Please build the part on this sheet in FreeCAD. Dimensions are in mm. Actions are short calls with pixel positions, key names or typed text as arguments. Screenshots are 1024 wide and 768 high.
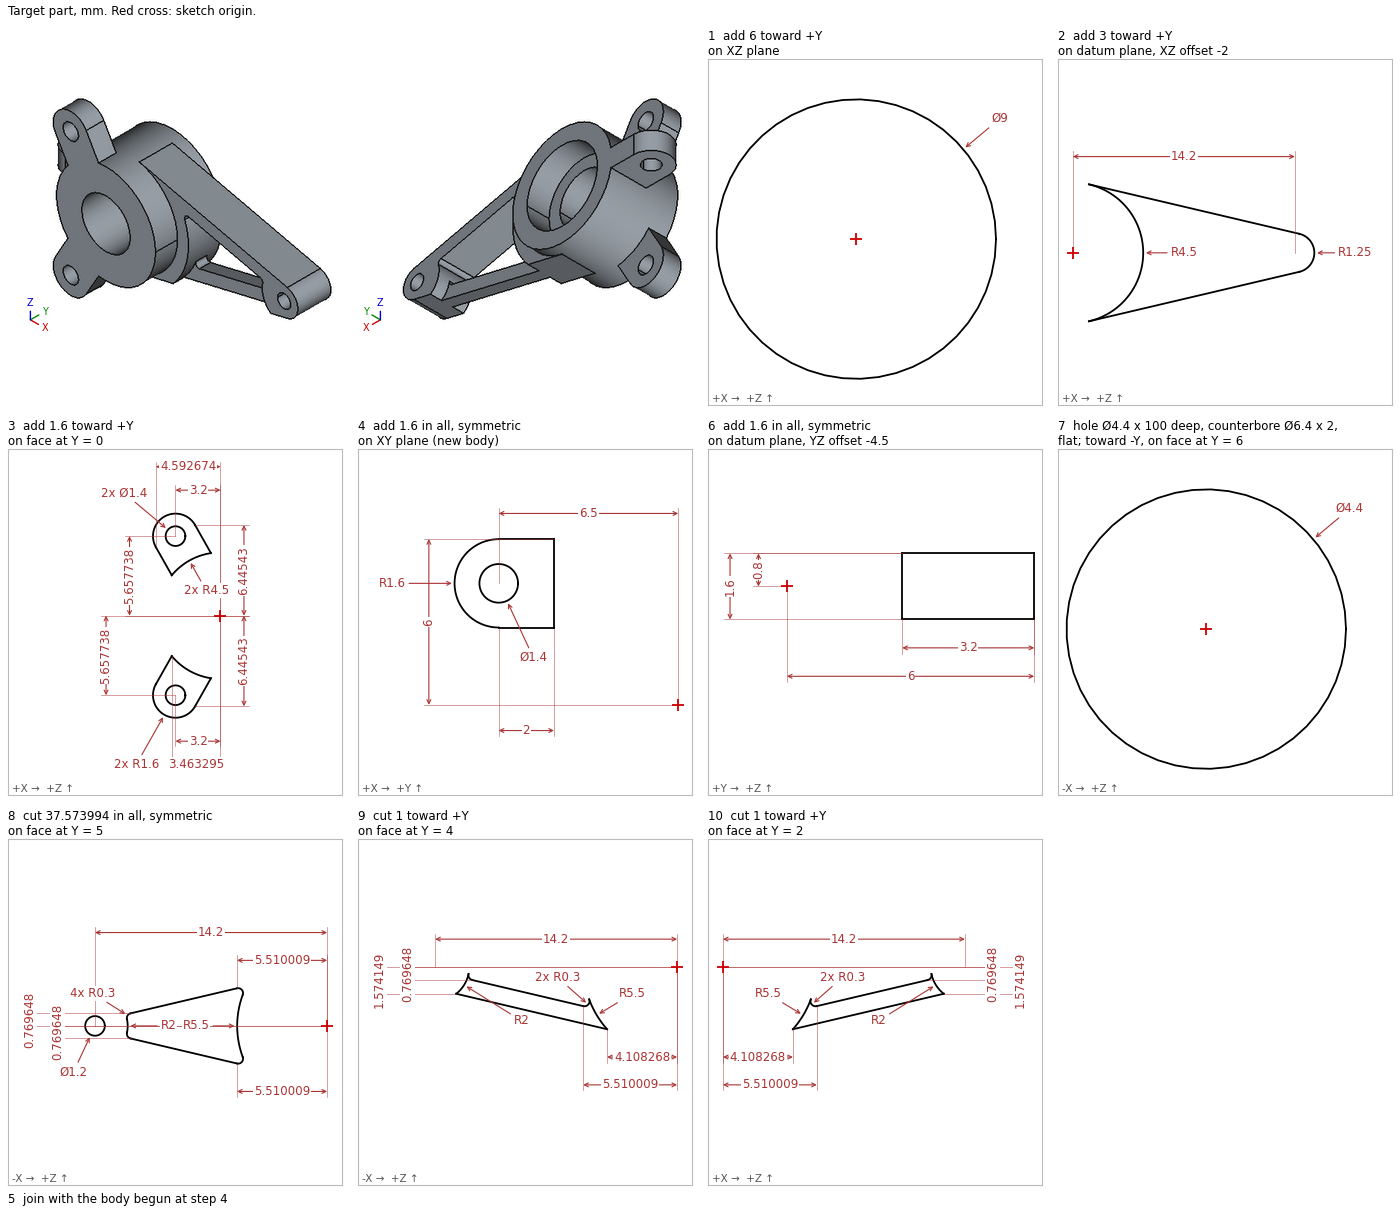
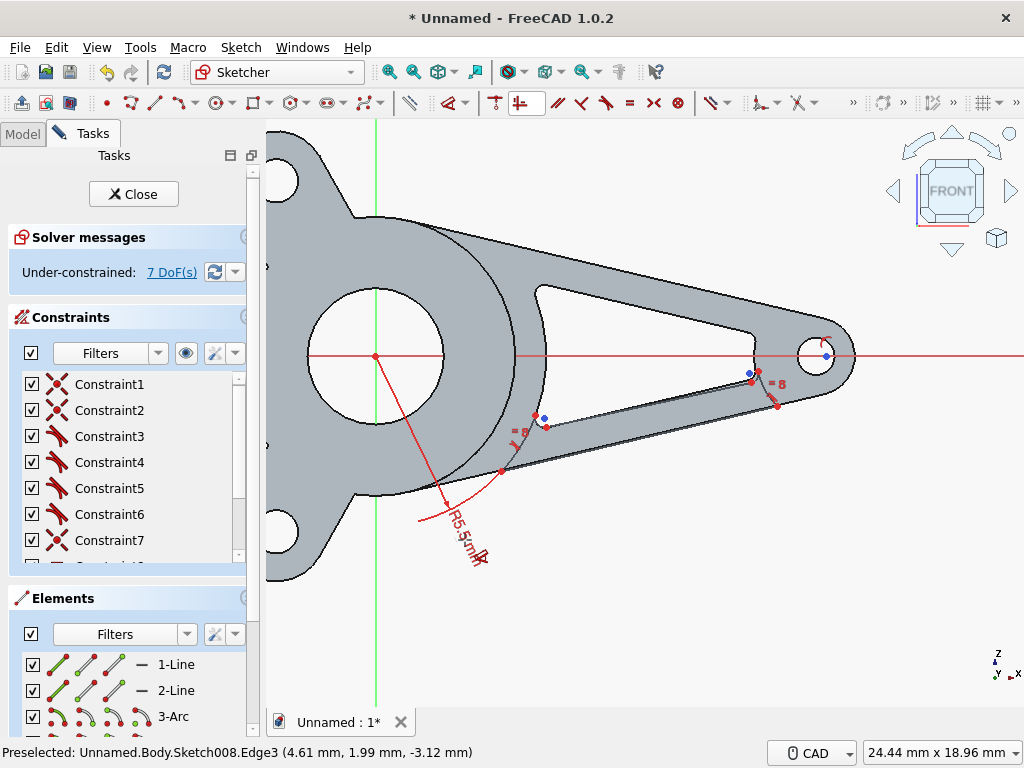
scroll(541, 427, up, 8)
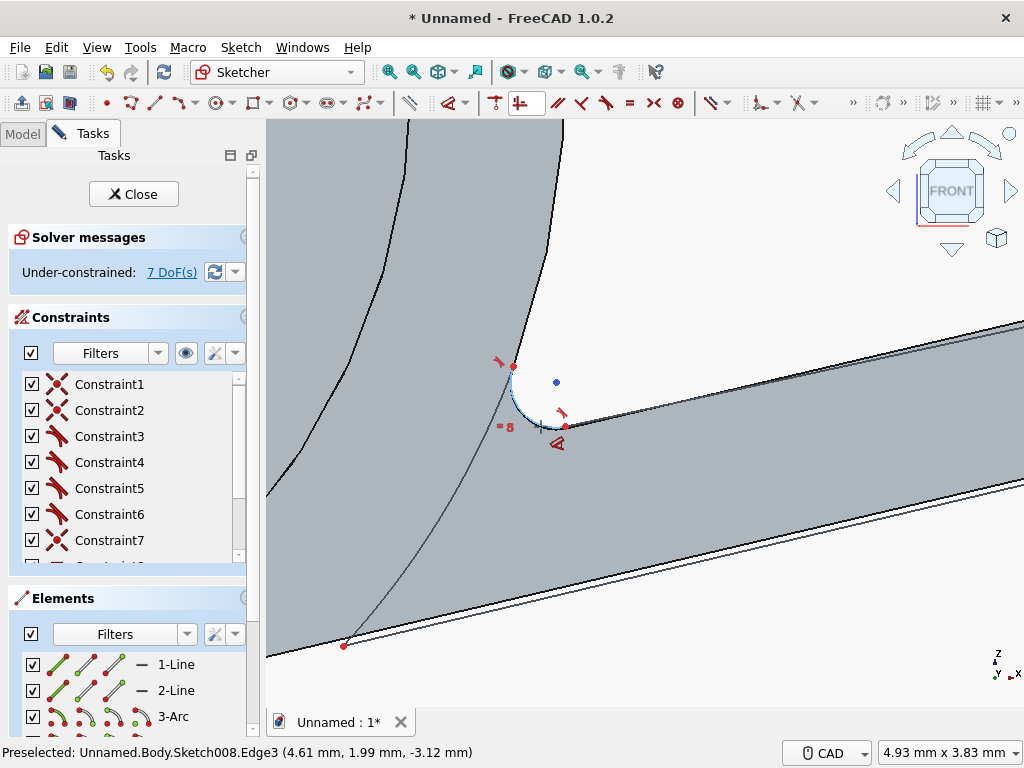
click(537, 424)
click(524, 453)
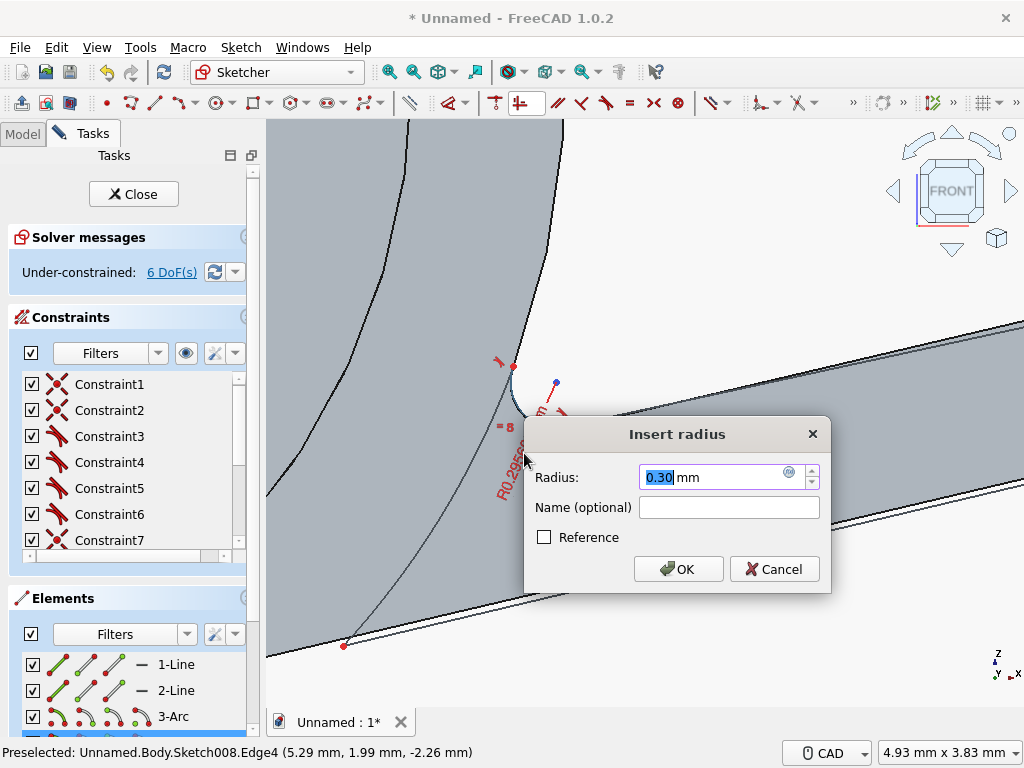
text(0.3)
key(Return)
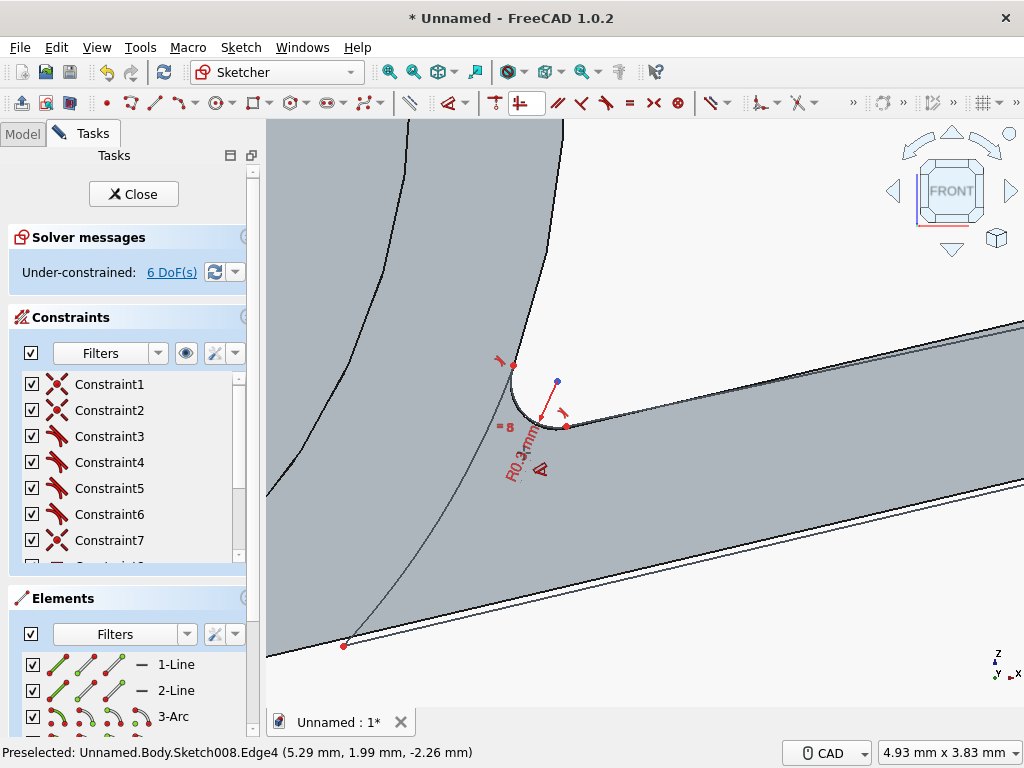
scroll(541, 427, down, 8)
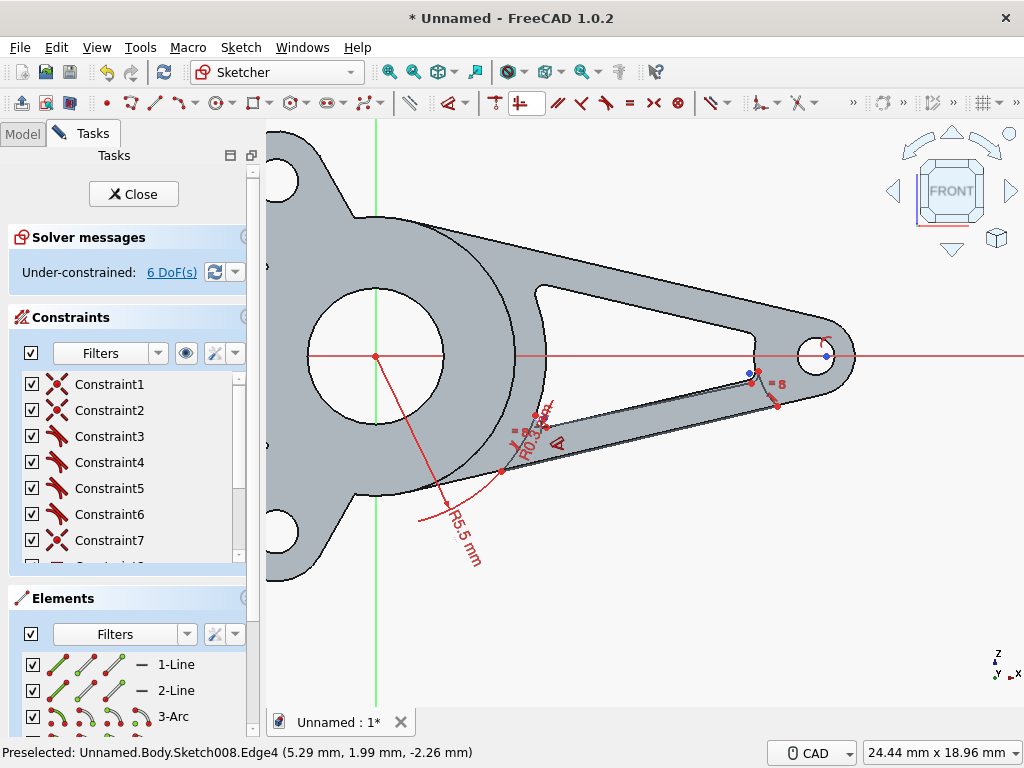
scroll(762, 383, up, 4)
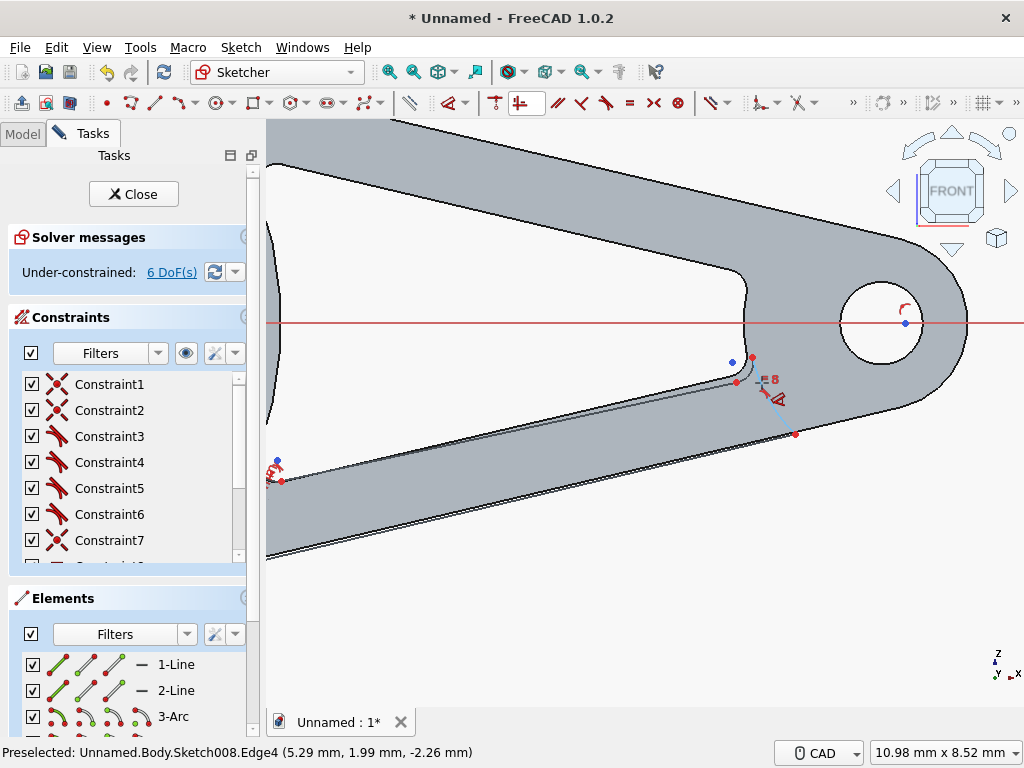
click(761, 383)
click(718, 303)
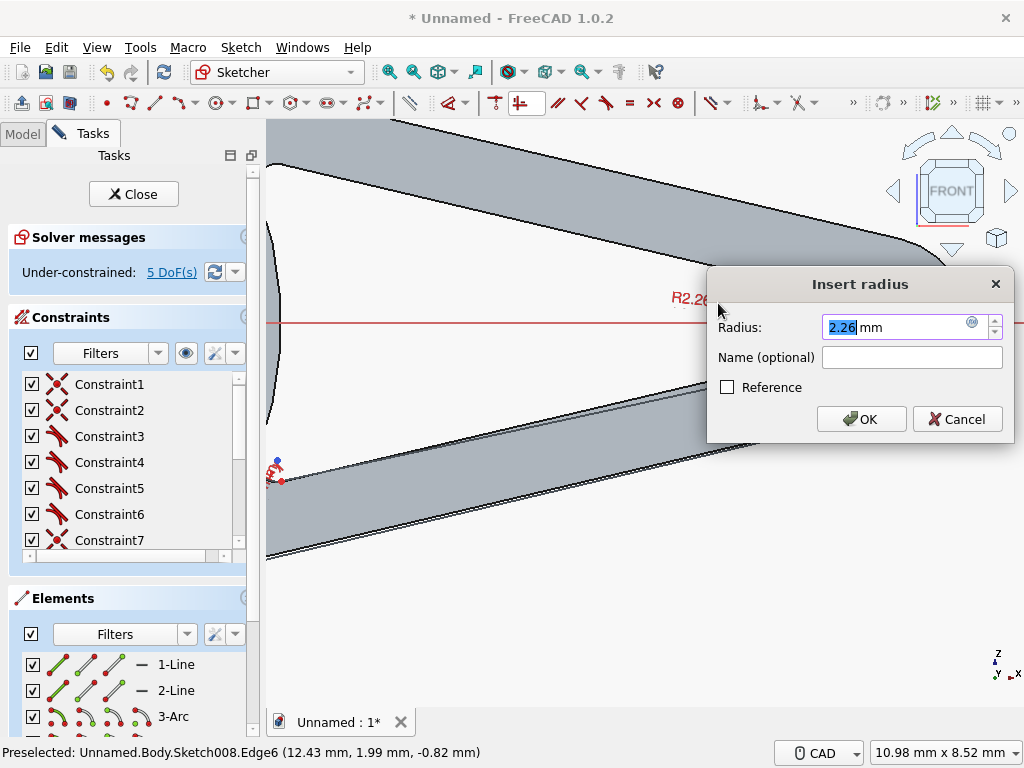
text(2)
key(Return)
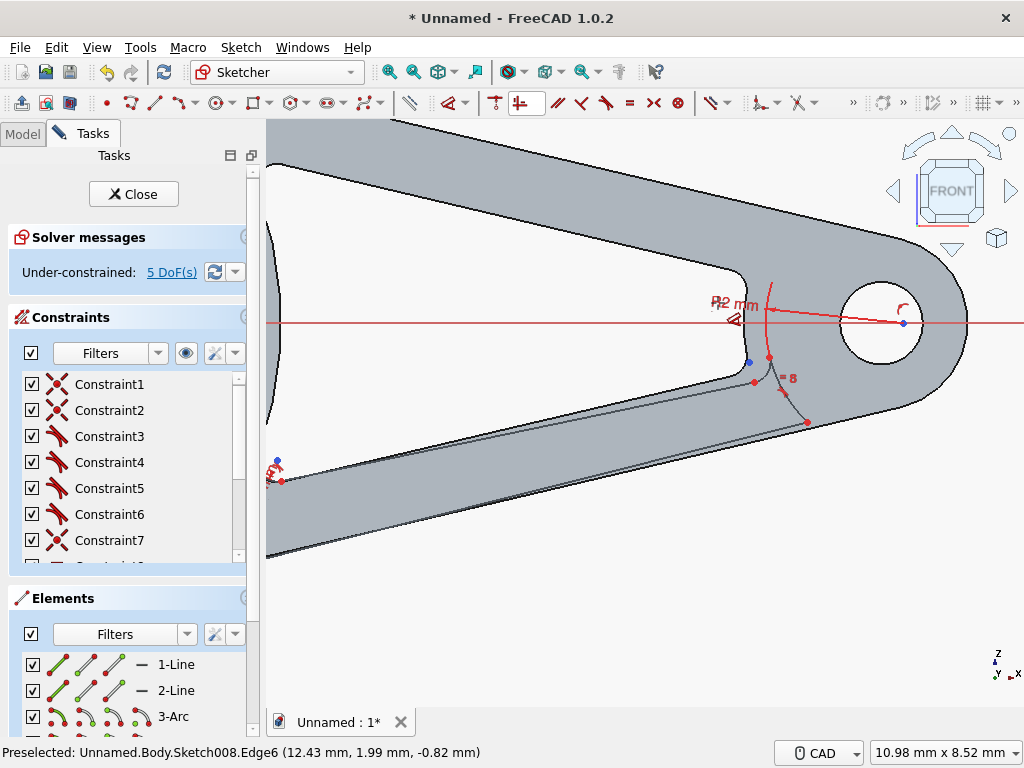
scroll(762, 383, down, 4)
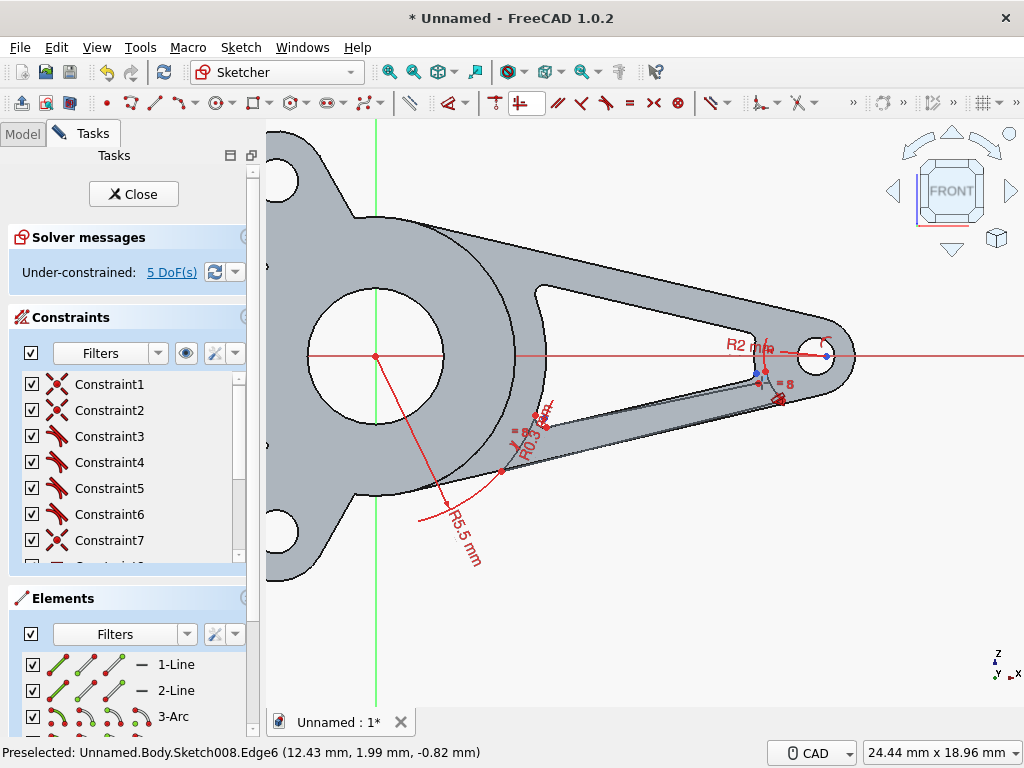
click(826, 356)
click(601, 322)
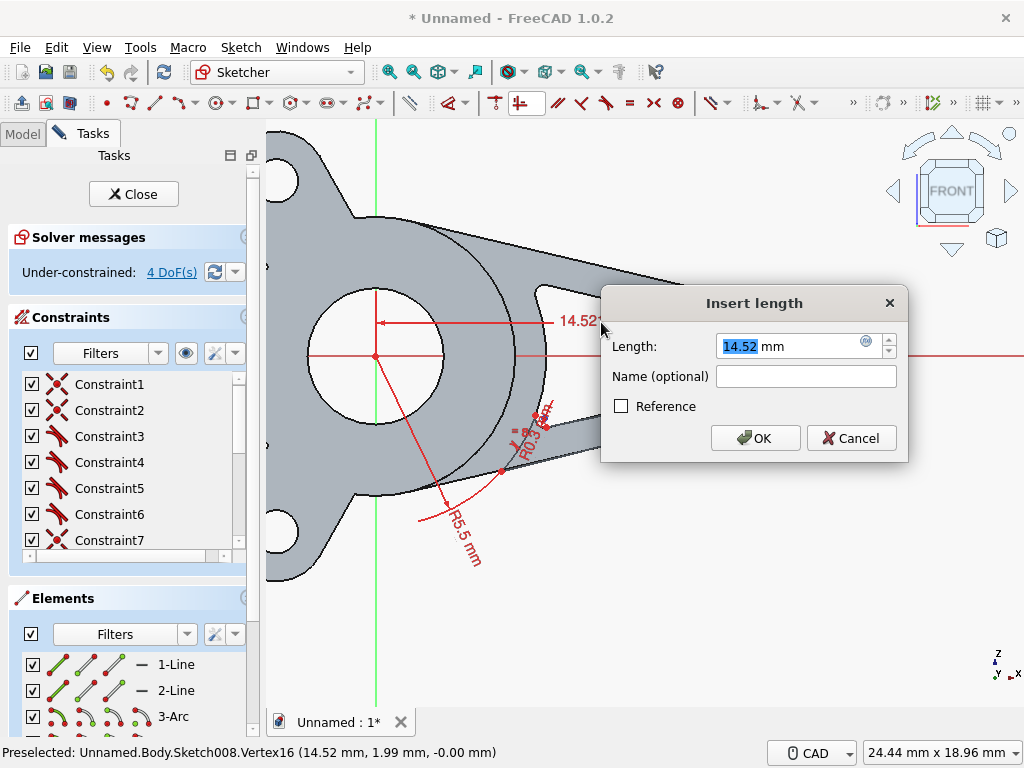
text(14.2)
key(Return)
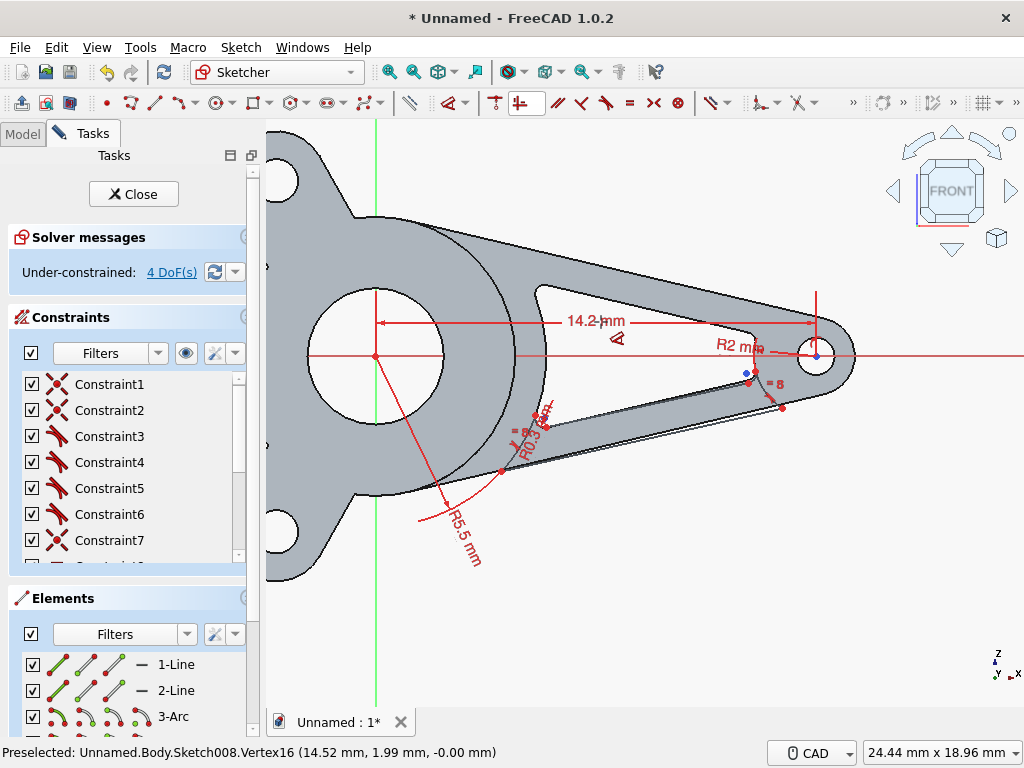
click(783, 409)
click(817, 382)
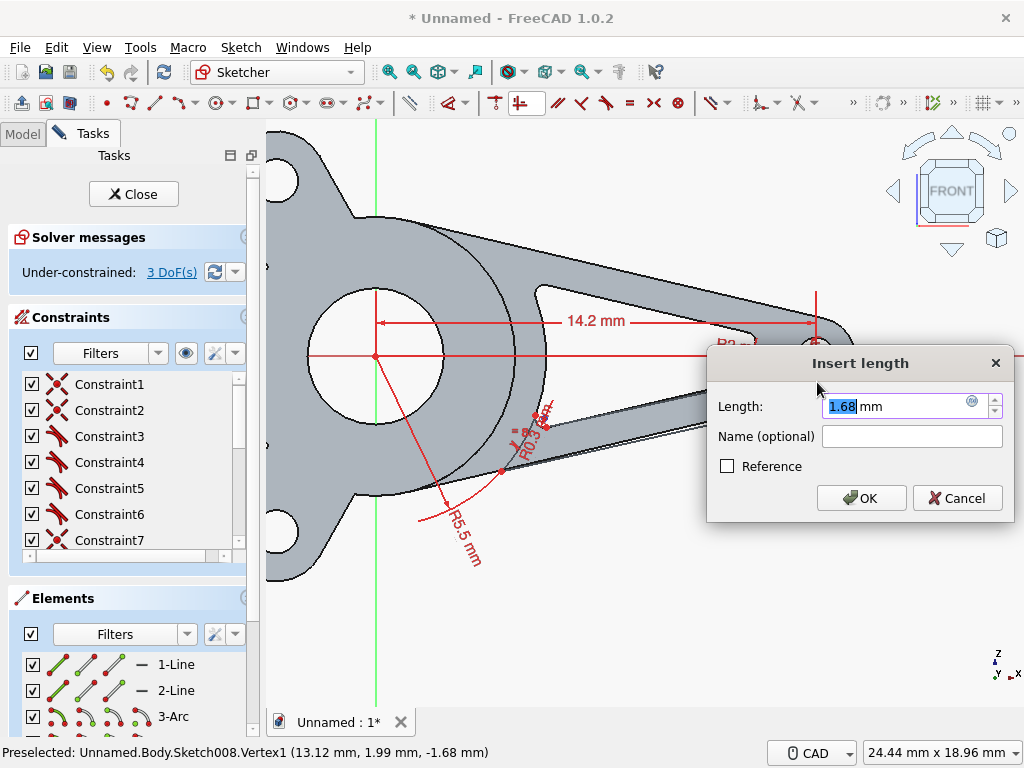
text(1.574149)
key(Return)